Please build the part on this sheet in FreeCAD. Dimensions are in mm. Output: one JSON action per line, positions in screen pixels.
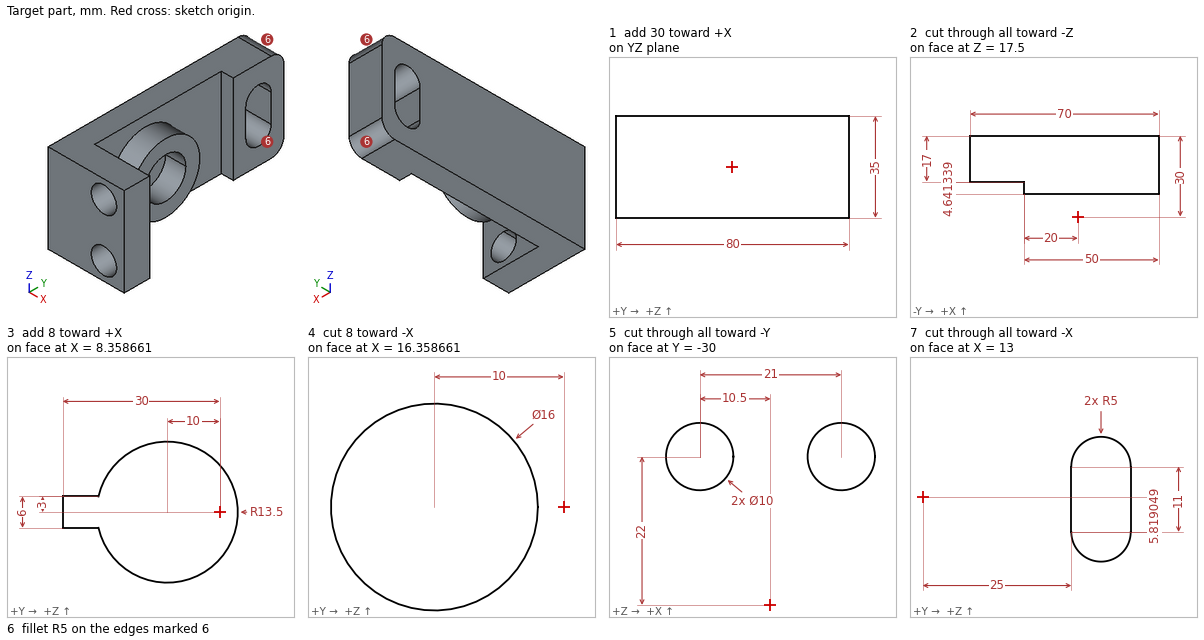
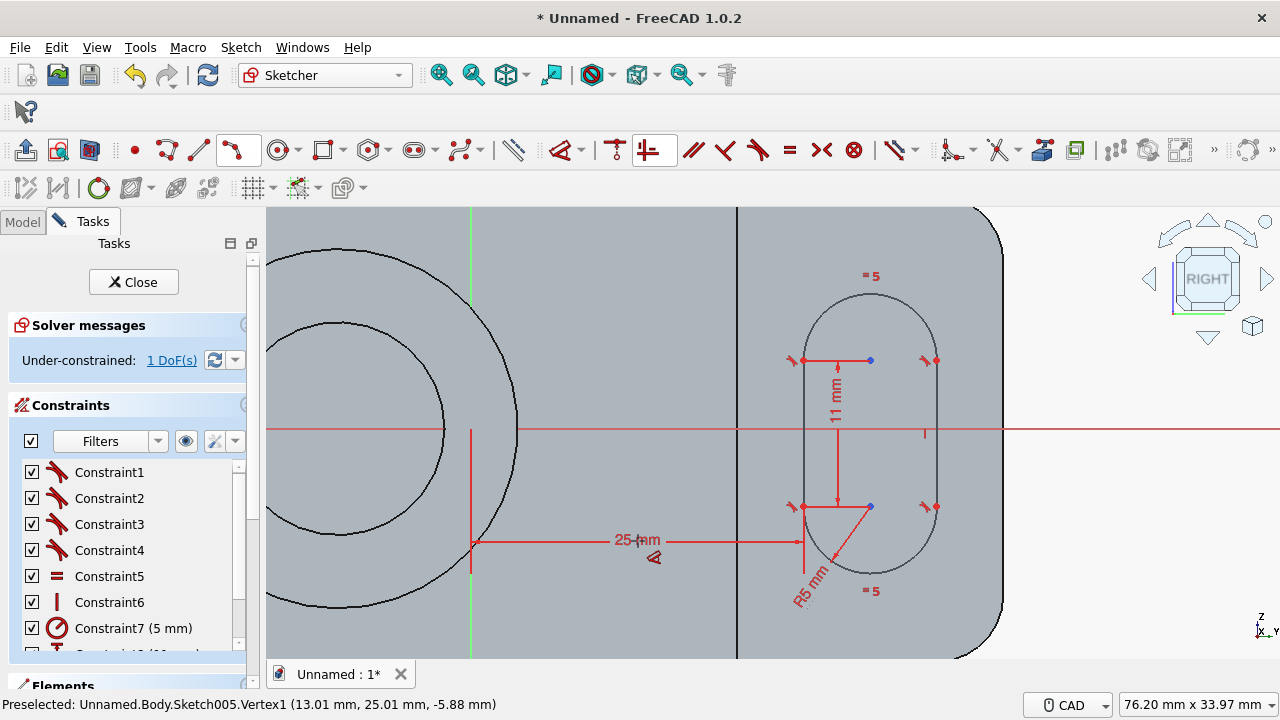
{"action": "left_click", "coordinate": [804, 507]}
{"action": "left_click", "coordinate": [437, 468]}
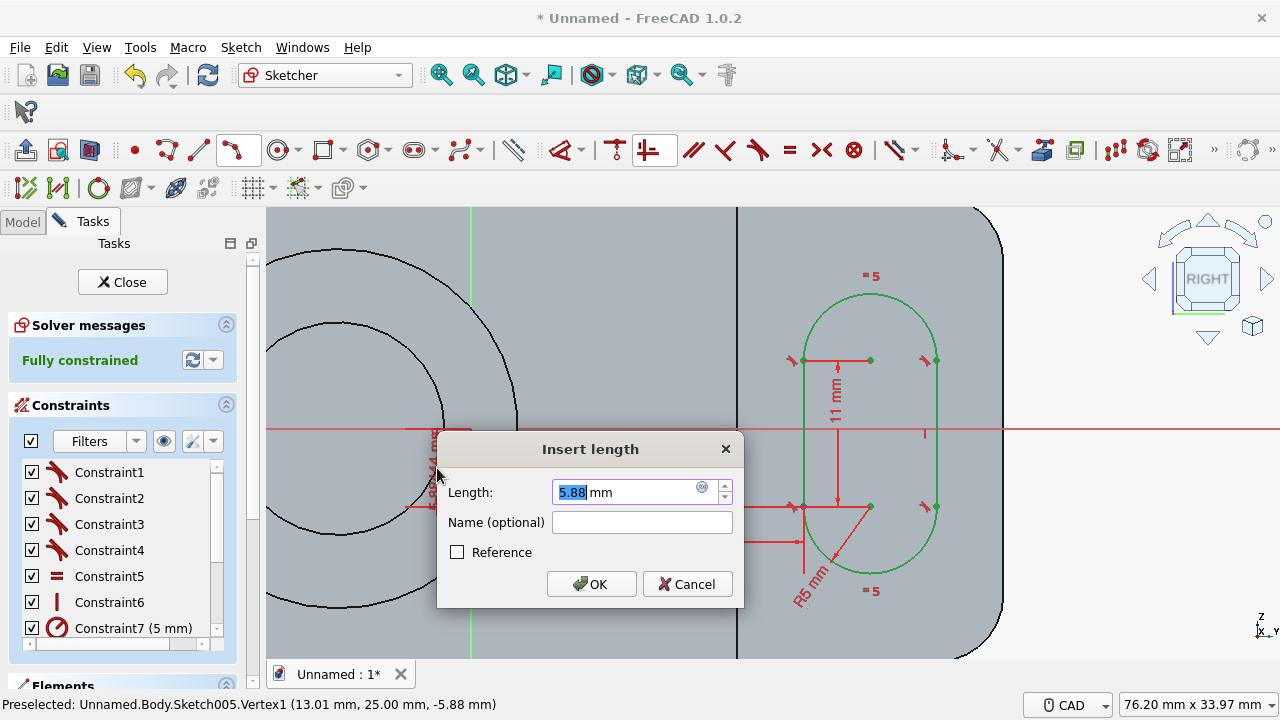
{"action": "type", "text": "5.819049"}
{"action": "key", "text": "Return"}
{"action": "key", "text": "Escape"}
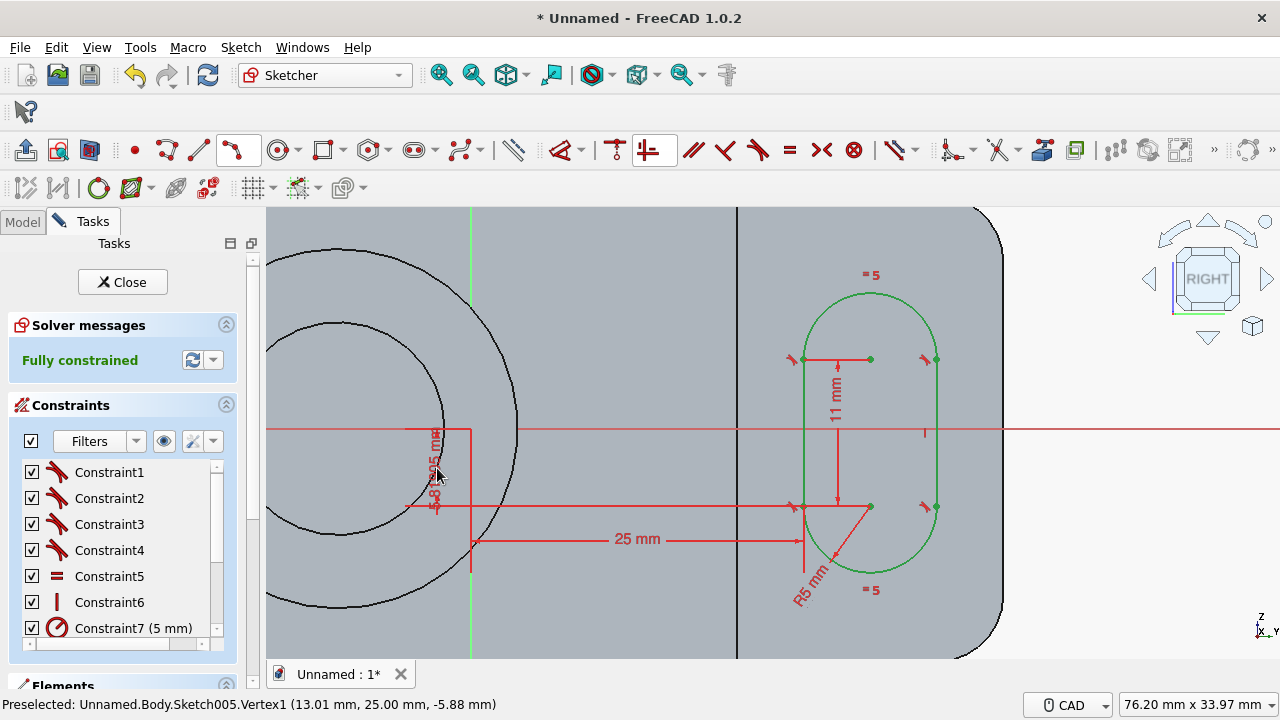
{"action": "left_click", "coordinate": [123, 282]}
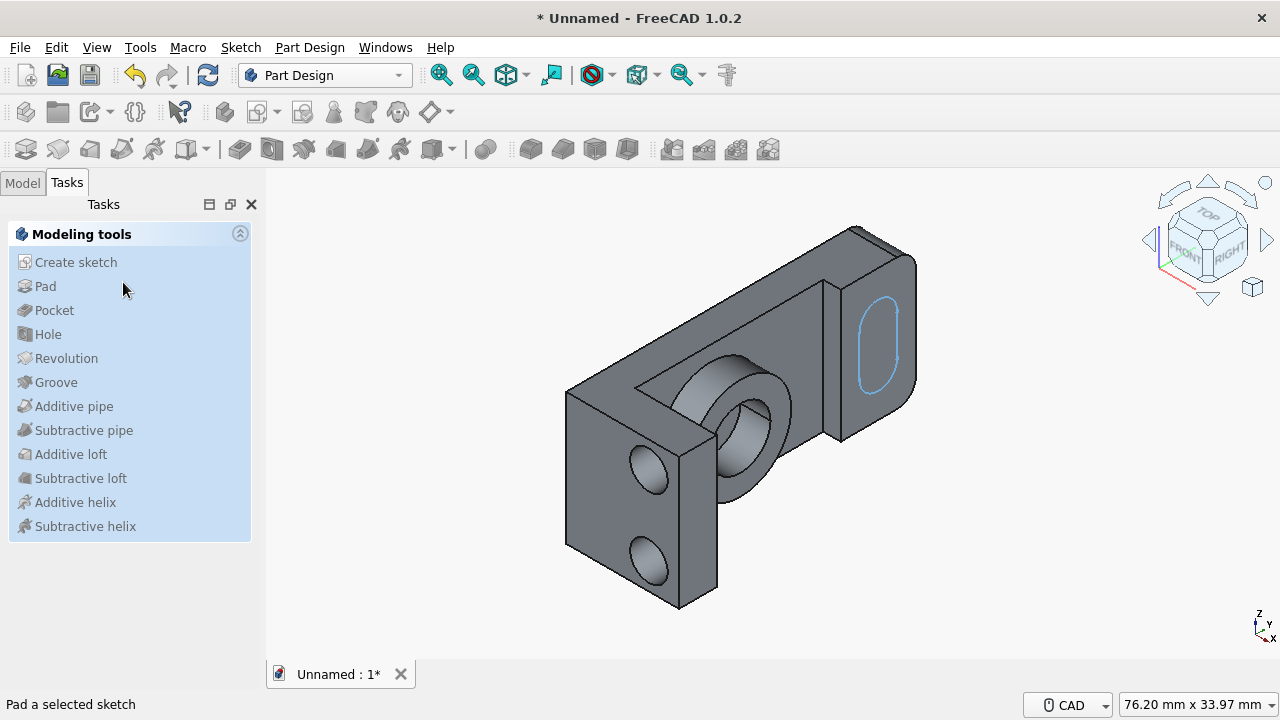
{"action": "left_click", "coordinate": [240, 150]}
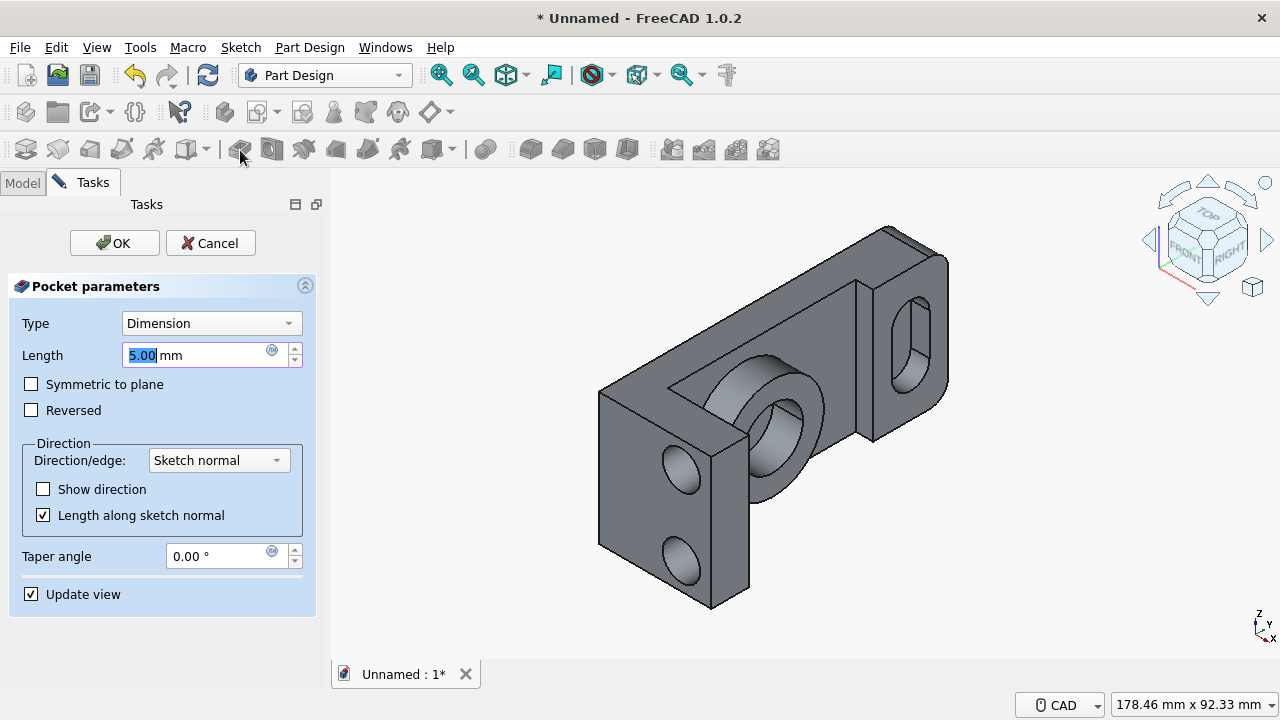
{"action": "left_click", "coordinate": [212, 324]}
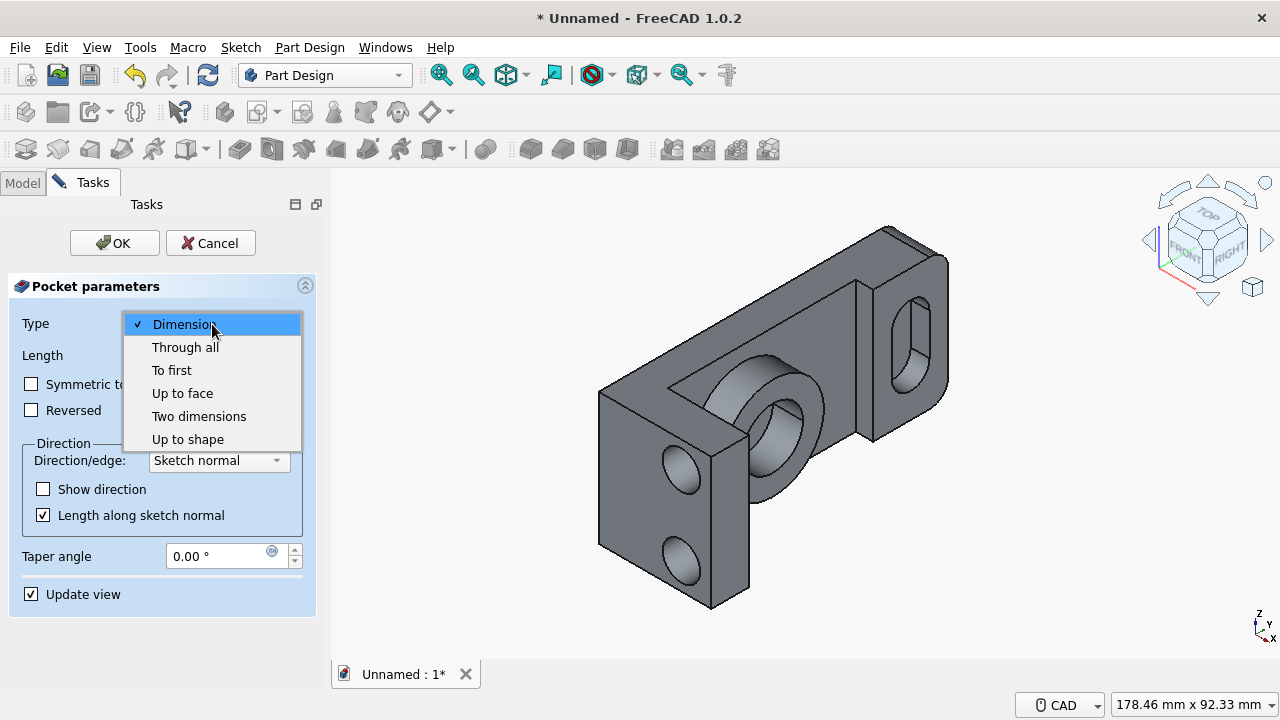
{"action": "left_click", "coordinate": [212, 348]}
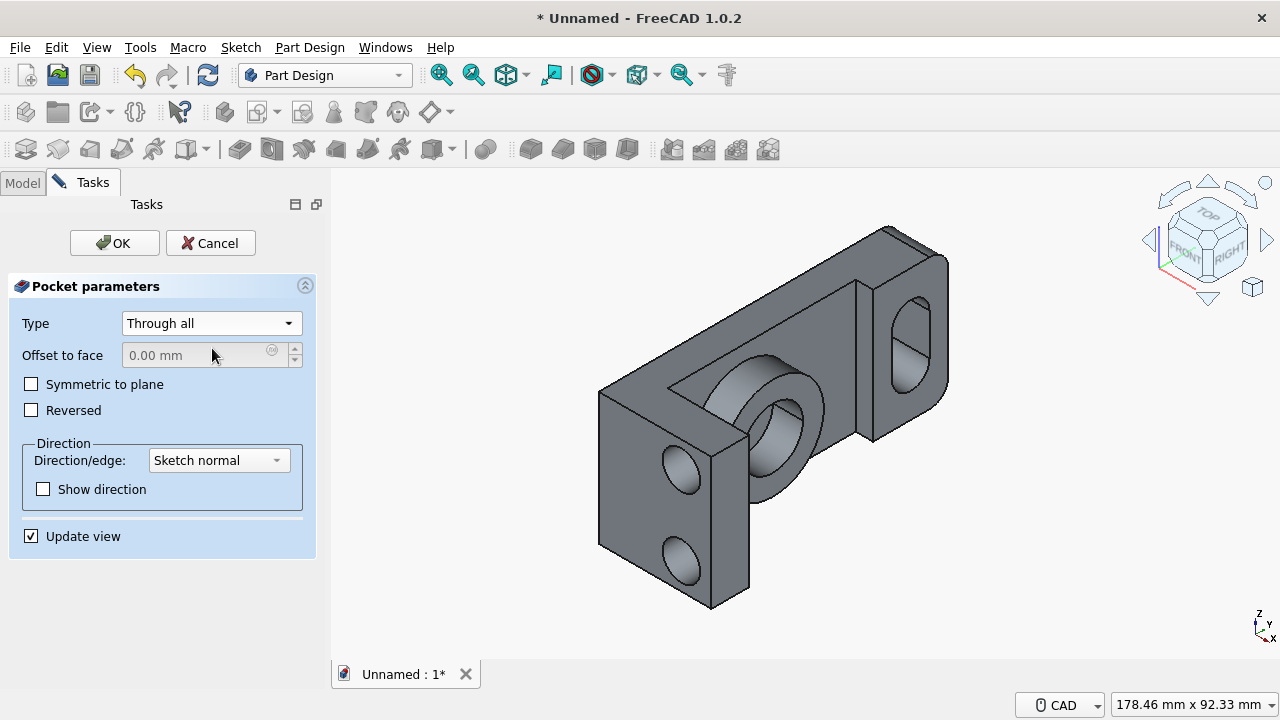
{"action": "left_click", "coordinate": [115, 243]}